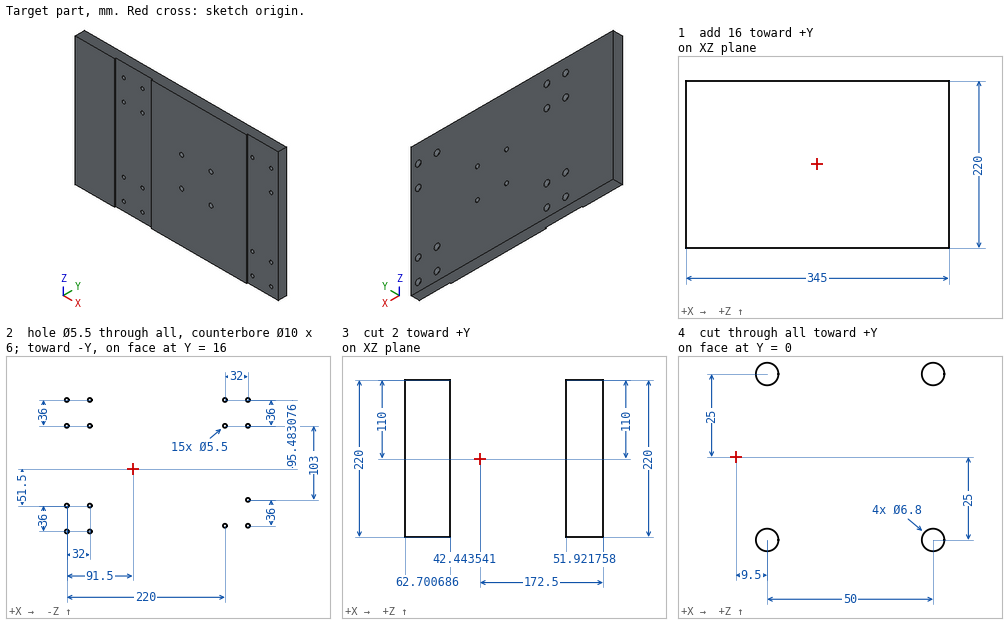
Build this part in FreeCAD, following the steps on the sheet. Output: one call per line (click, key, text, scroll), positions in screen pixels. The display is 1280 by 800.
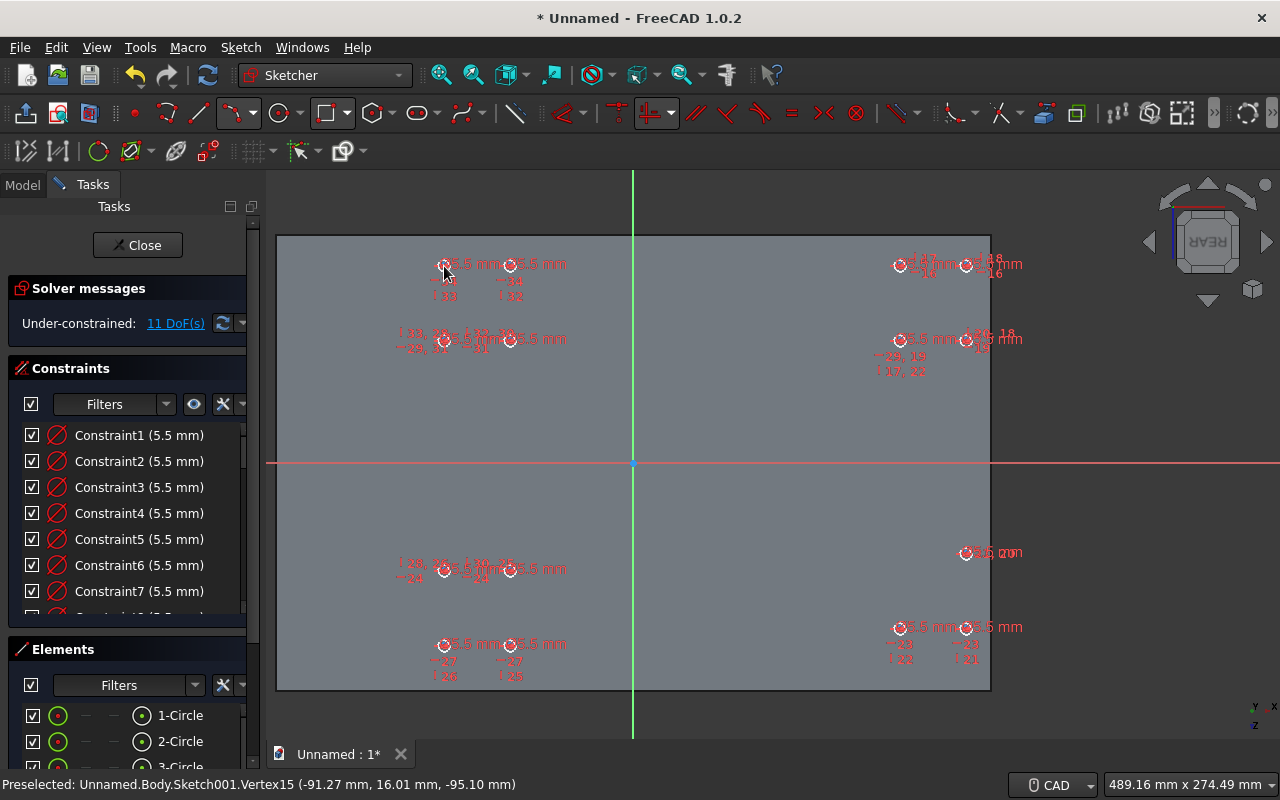
click(562, 114)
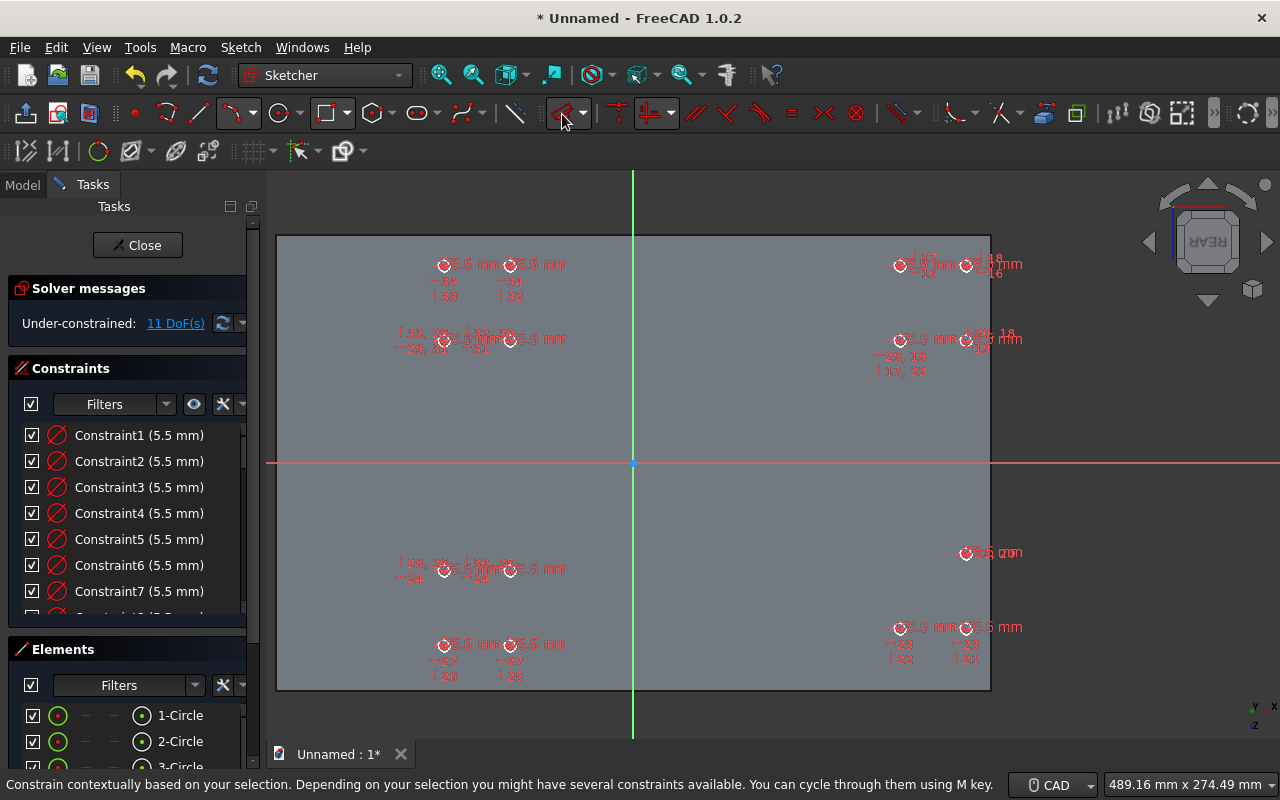
click(966, 266)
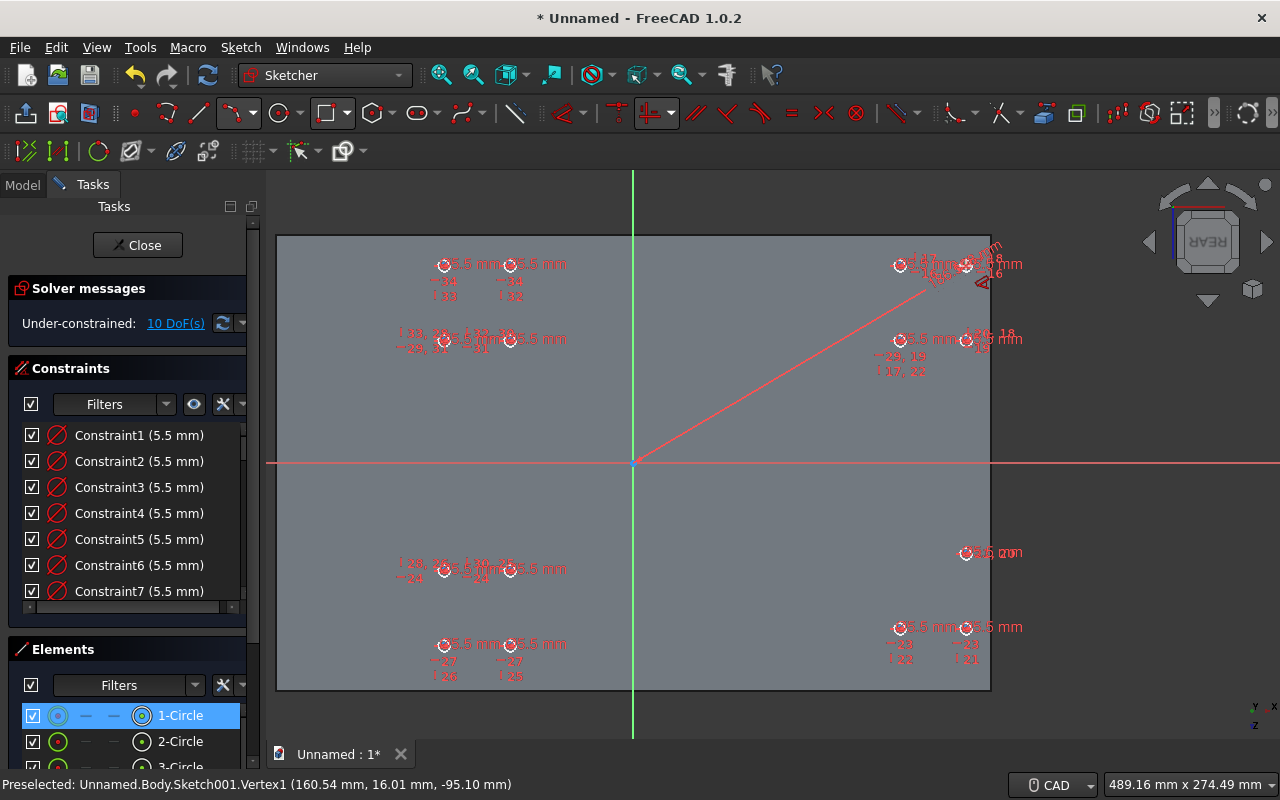
click(900, 266)
click(933, 232)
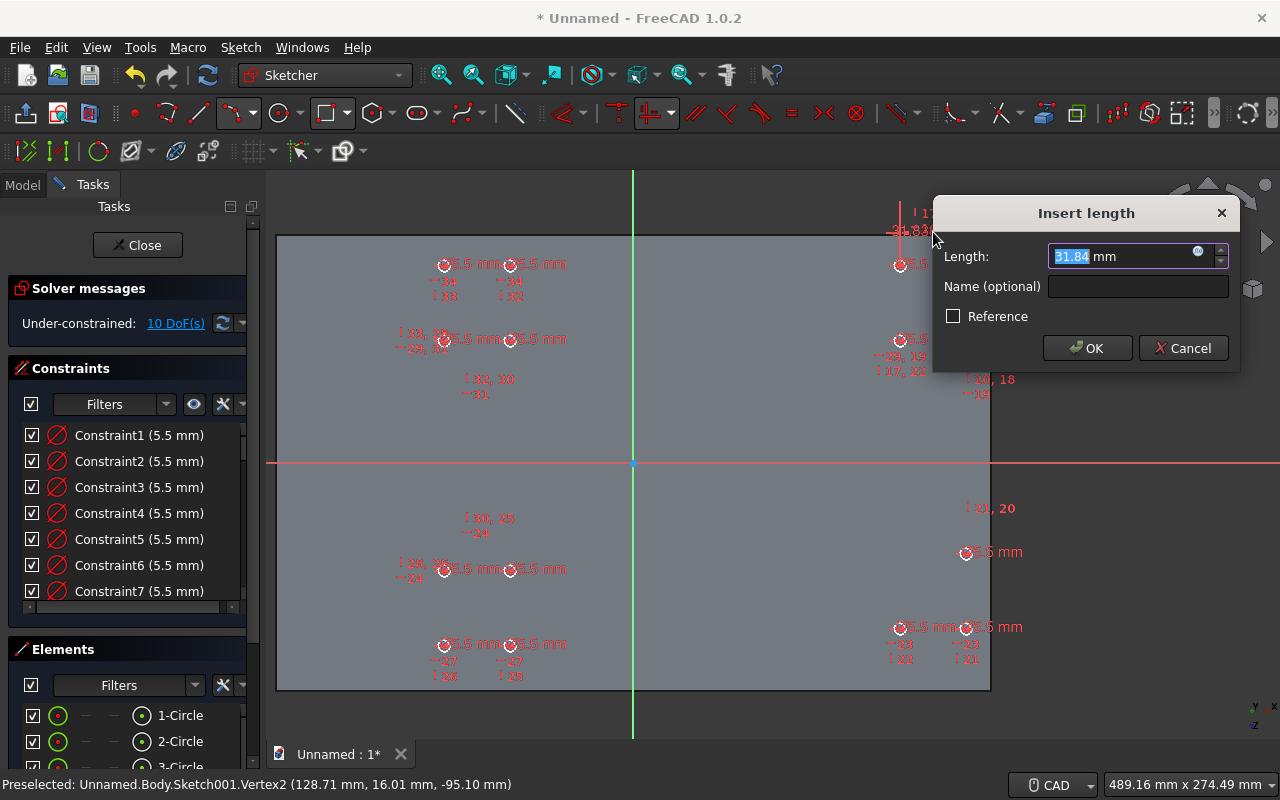
text(32)
key(Return)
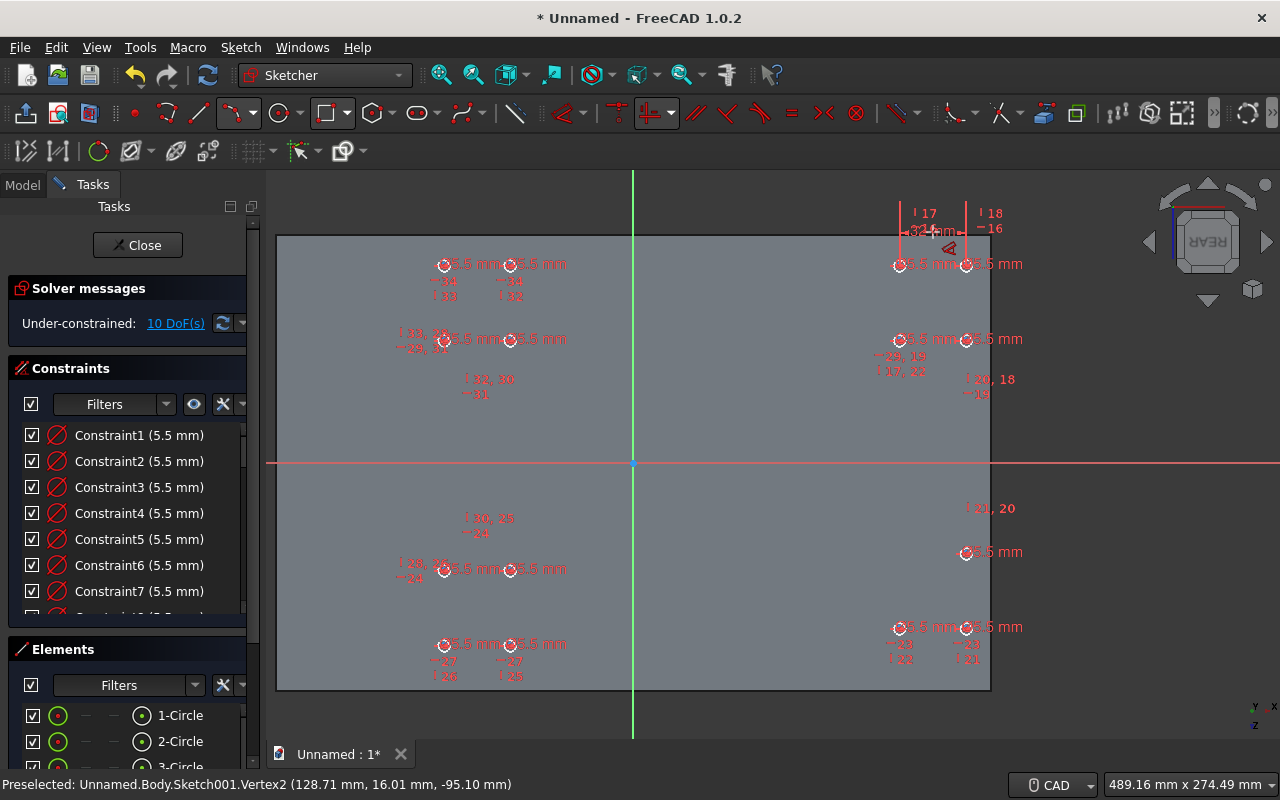
click(900, 266)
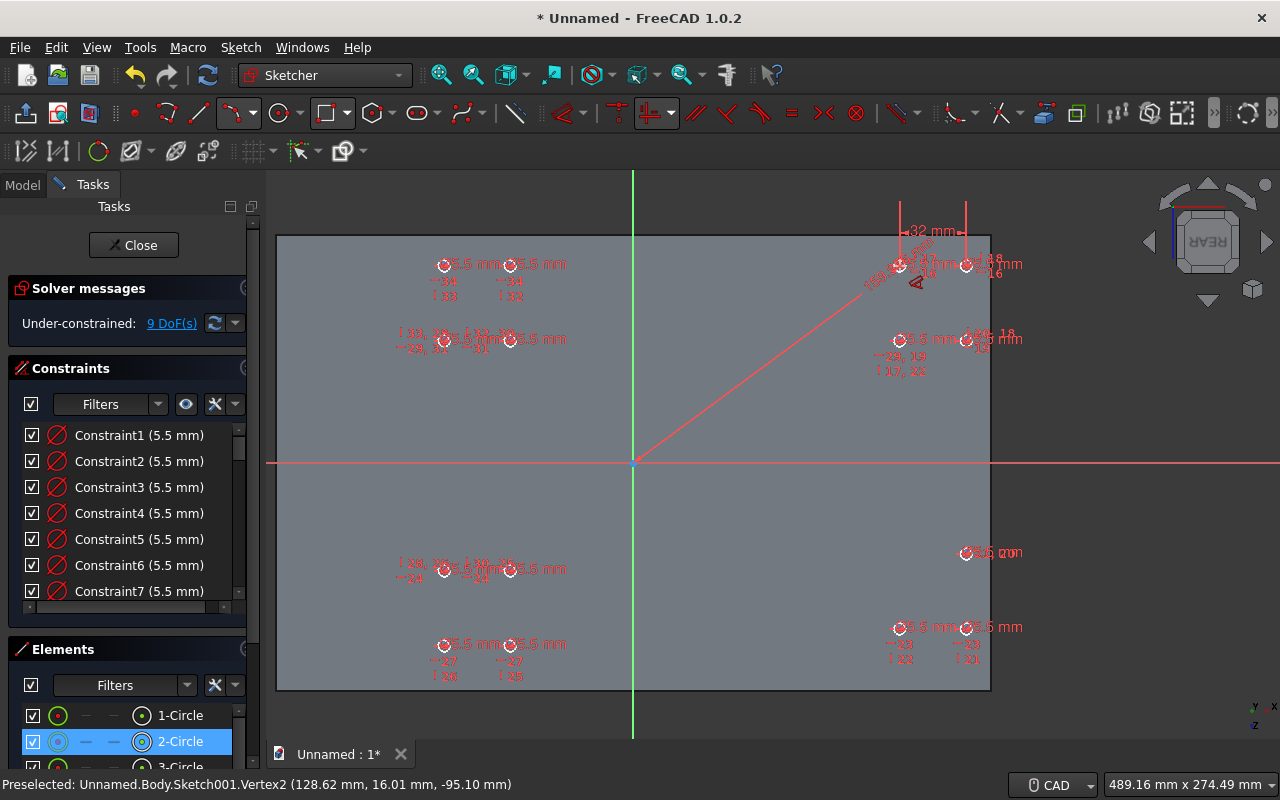
click(900, 341)
click(934, 303)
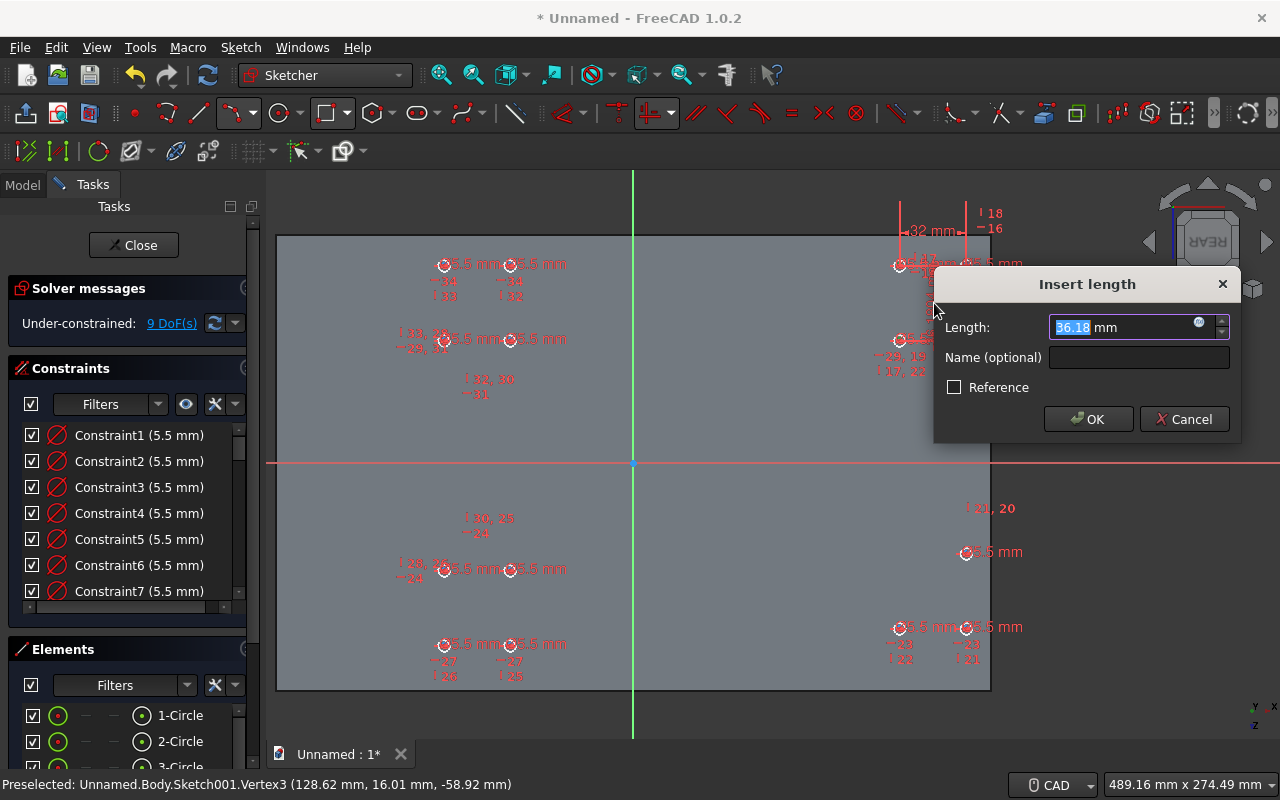
text(36)
key(Return)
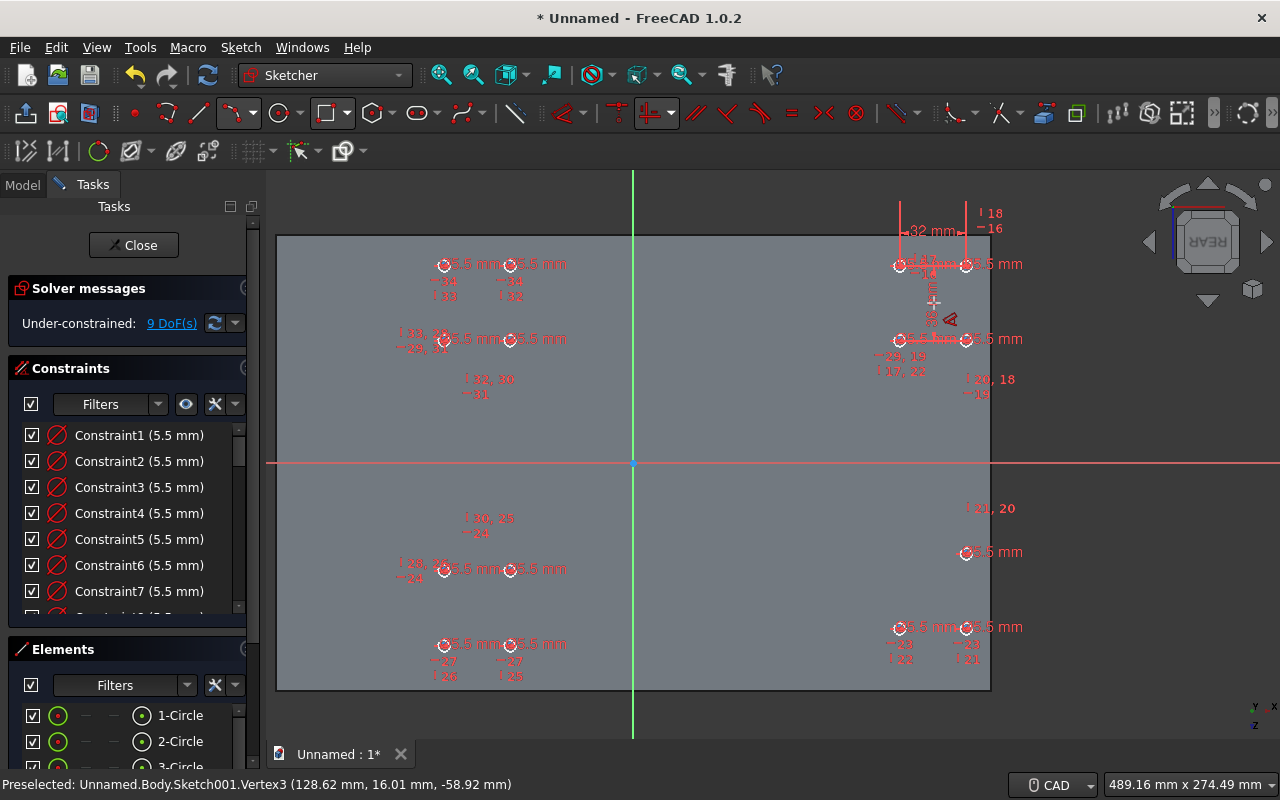
click(966, 554)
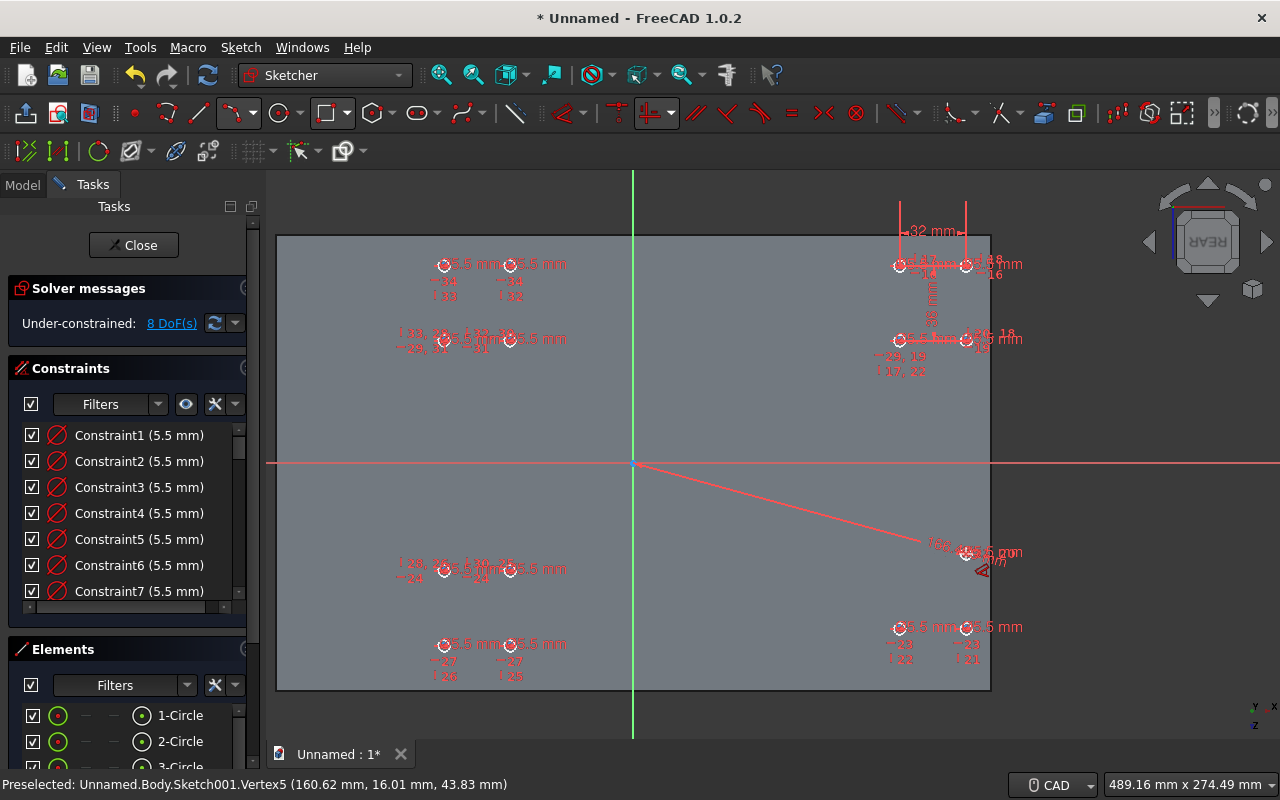
click(966, 629)
click(1000, 591)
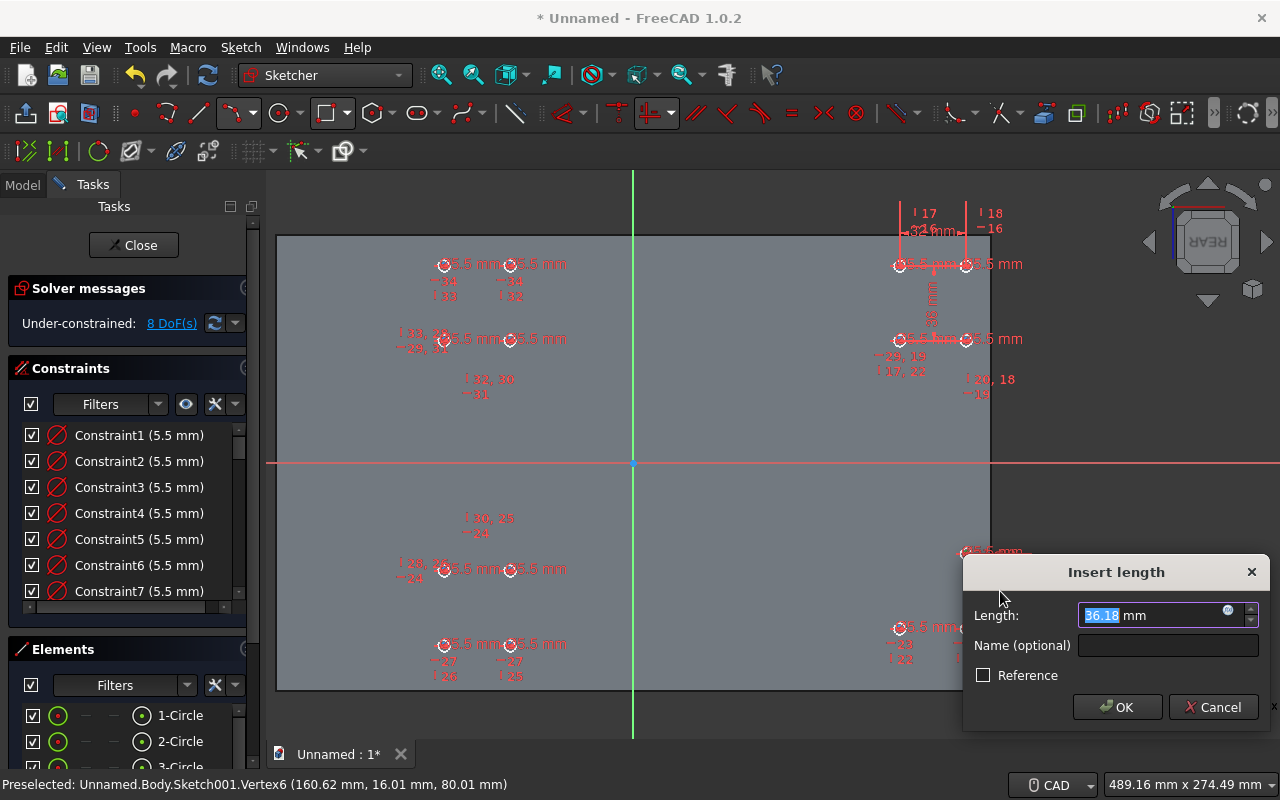
text(36)
key(Return)